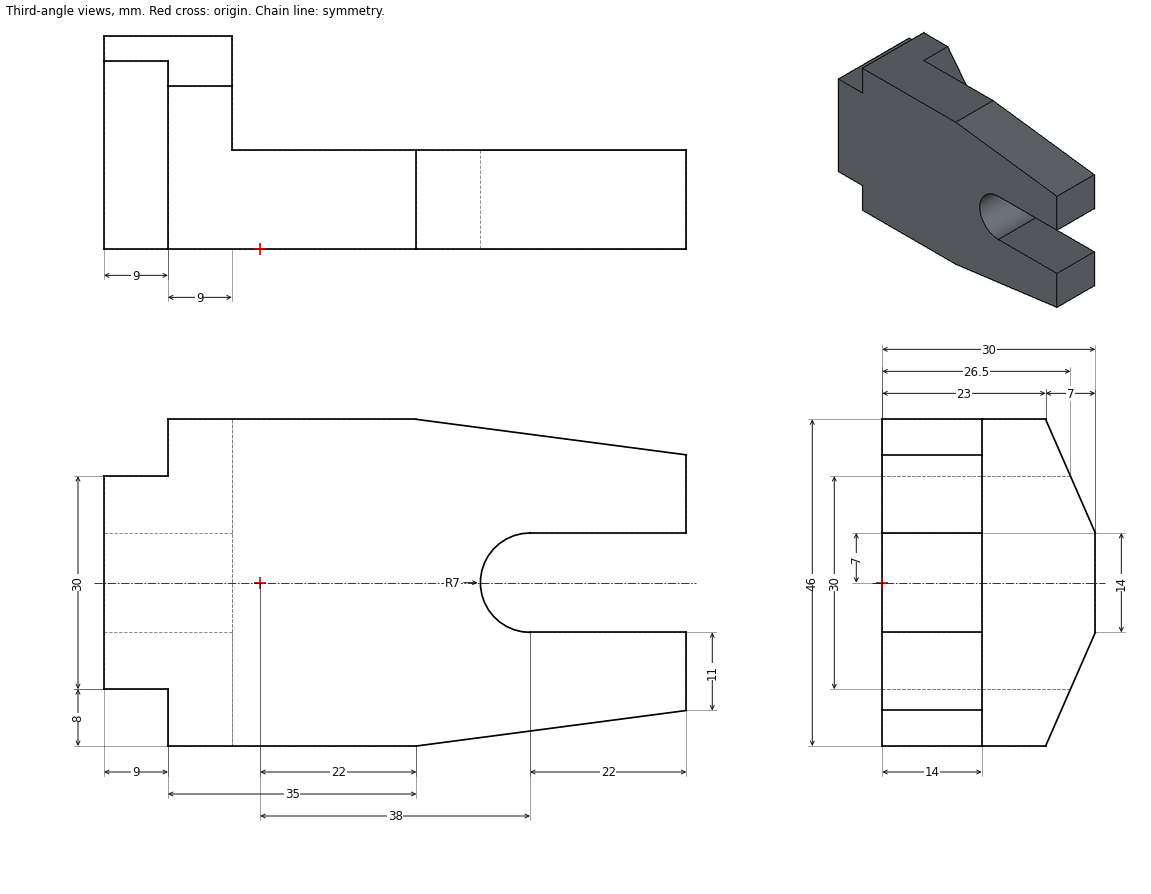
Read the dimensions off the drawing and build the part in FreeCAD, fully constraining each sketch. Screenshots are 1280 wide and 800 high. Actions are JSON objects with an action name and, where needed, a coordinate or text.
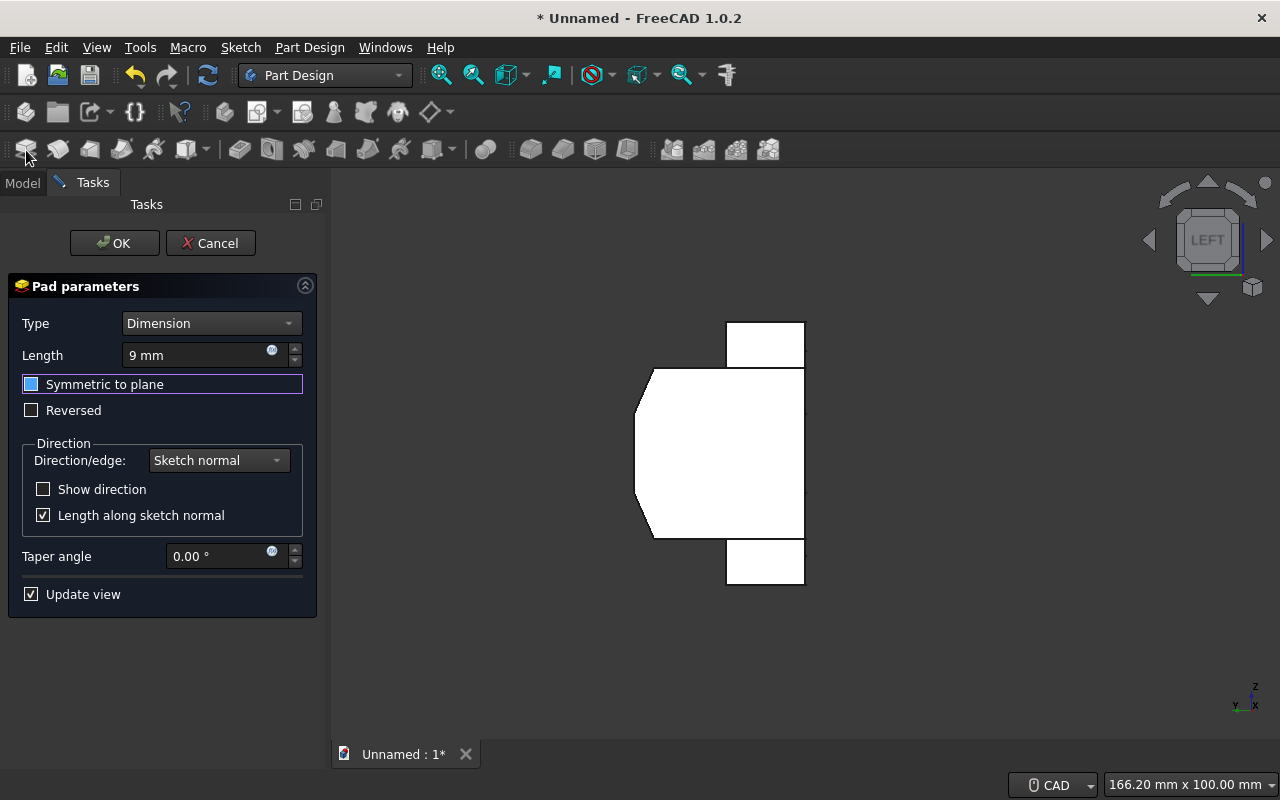
{"action": "left_click", "coordinate": [30, 410]}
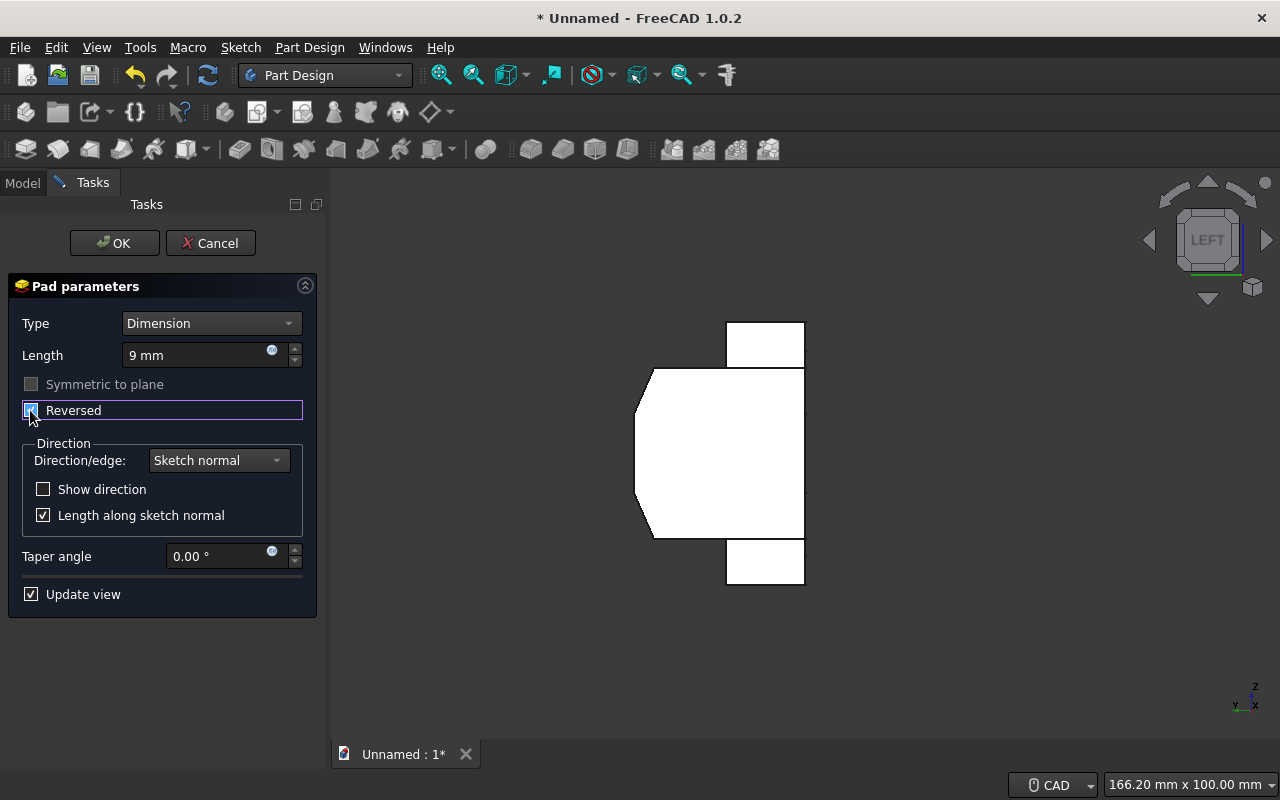
{"action": "left_click", "coordinate": [115, 243]}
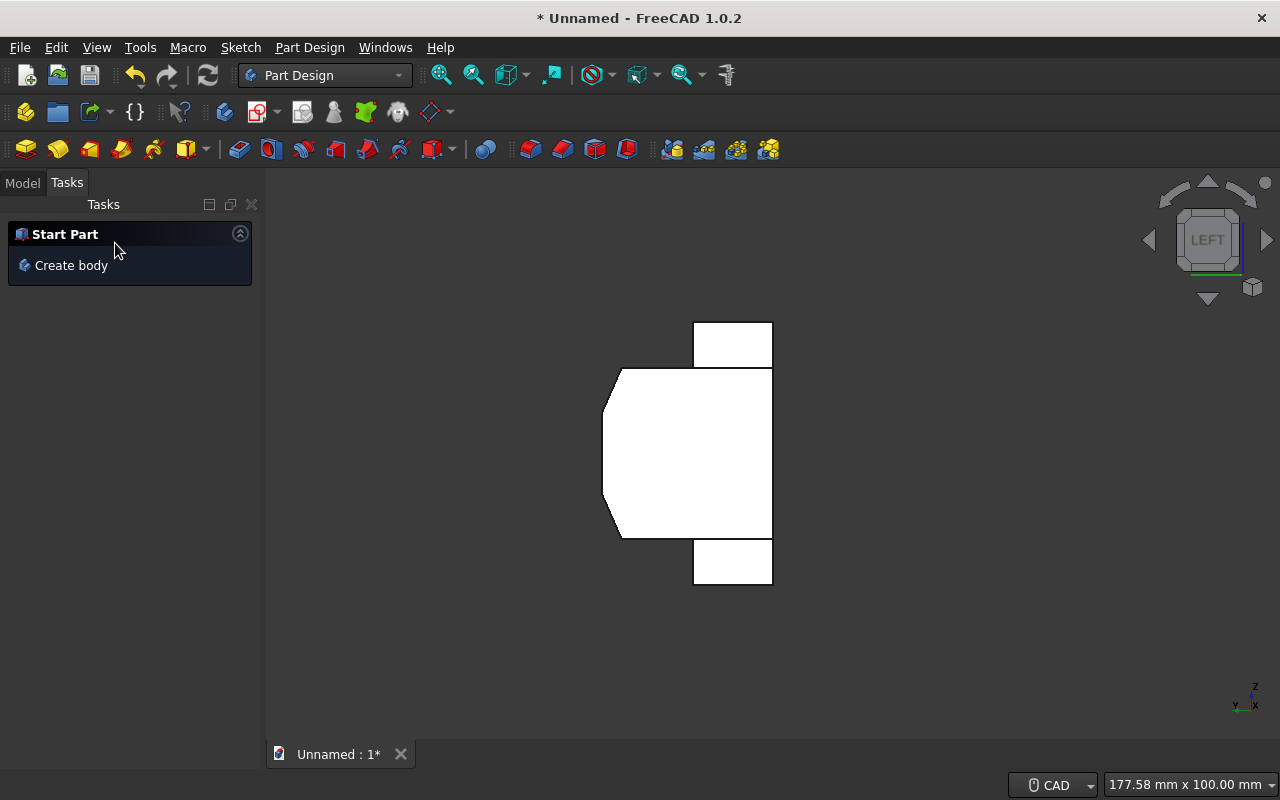
{"action": "key", "text": "0"}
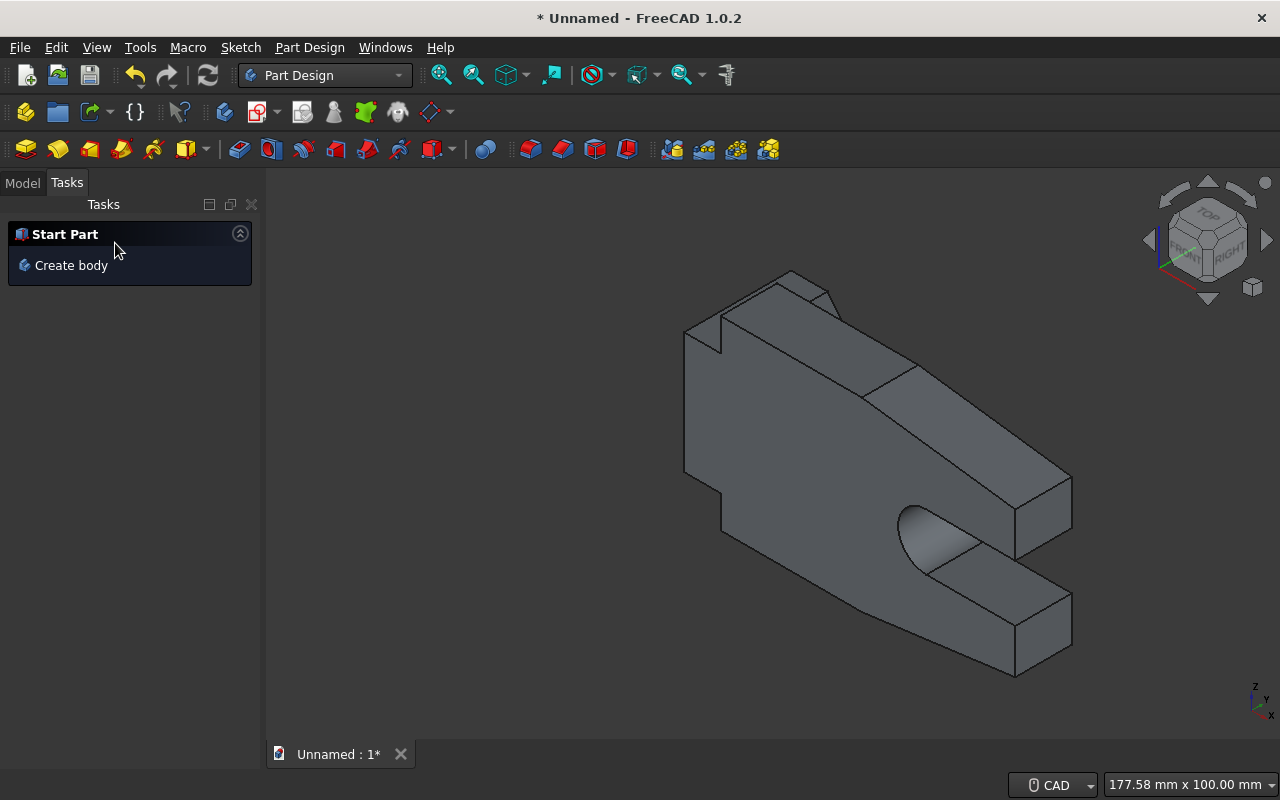
{"action": "key", "text": "3"}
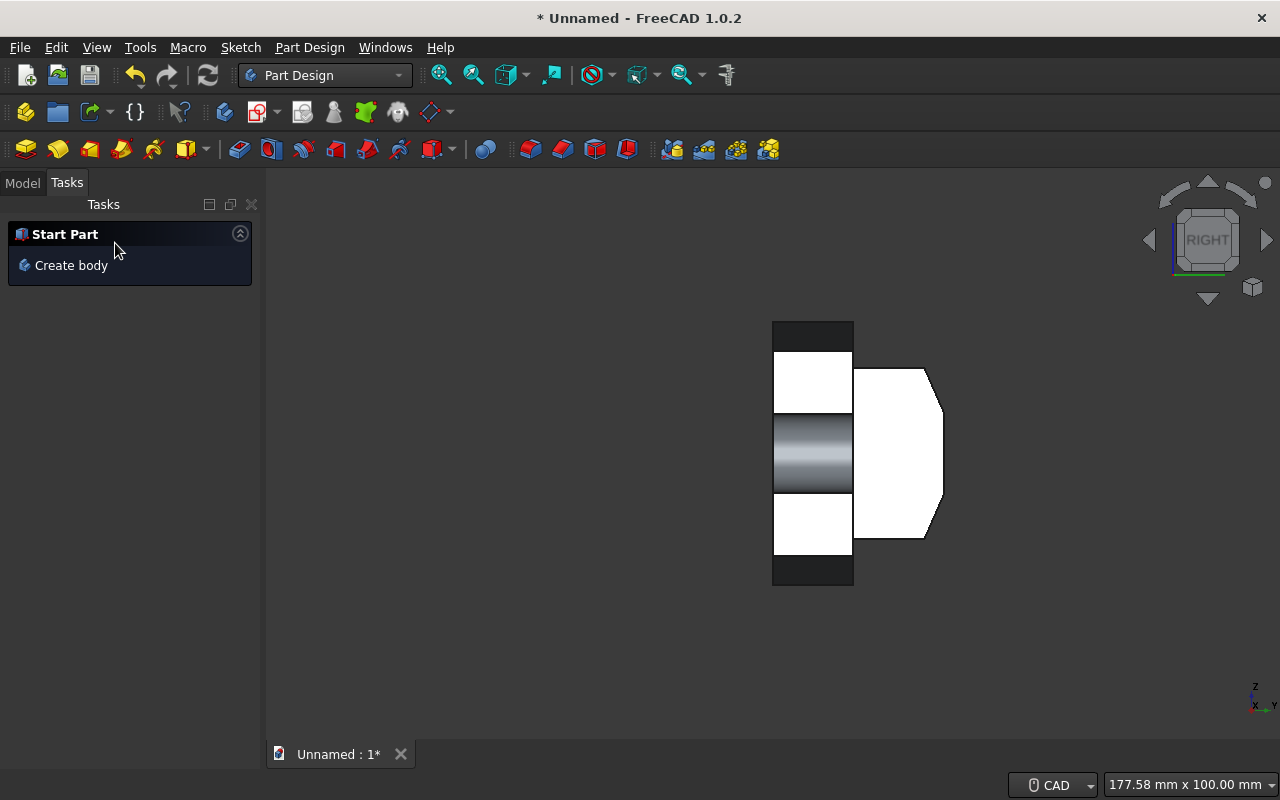
{"action": "left_click", "coordinate": [899, 428]}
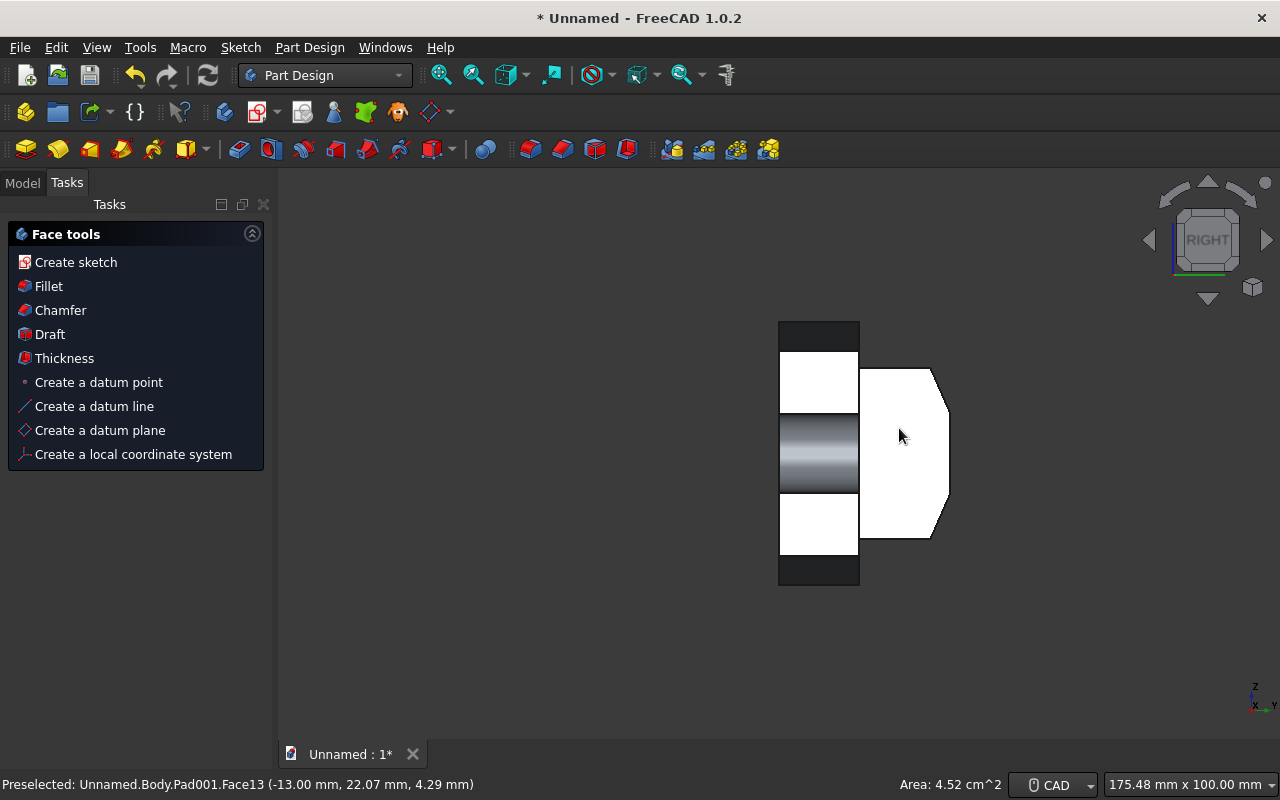
{"action": "left_click", "coordinate": [258, 112]}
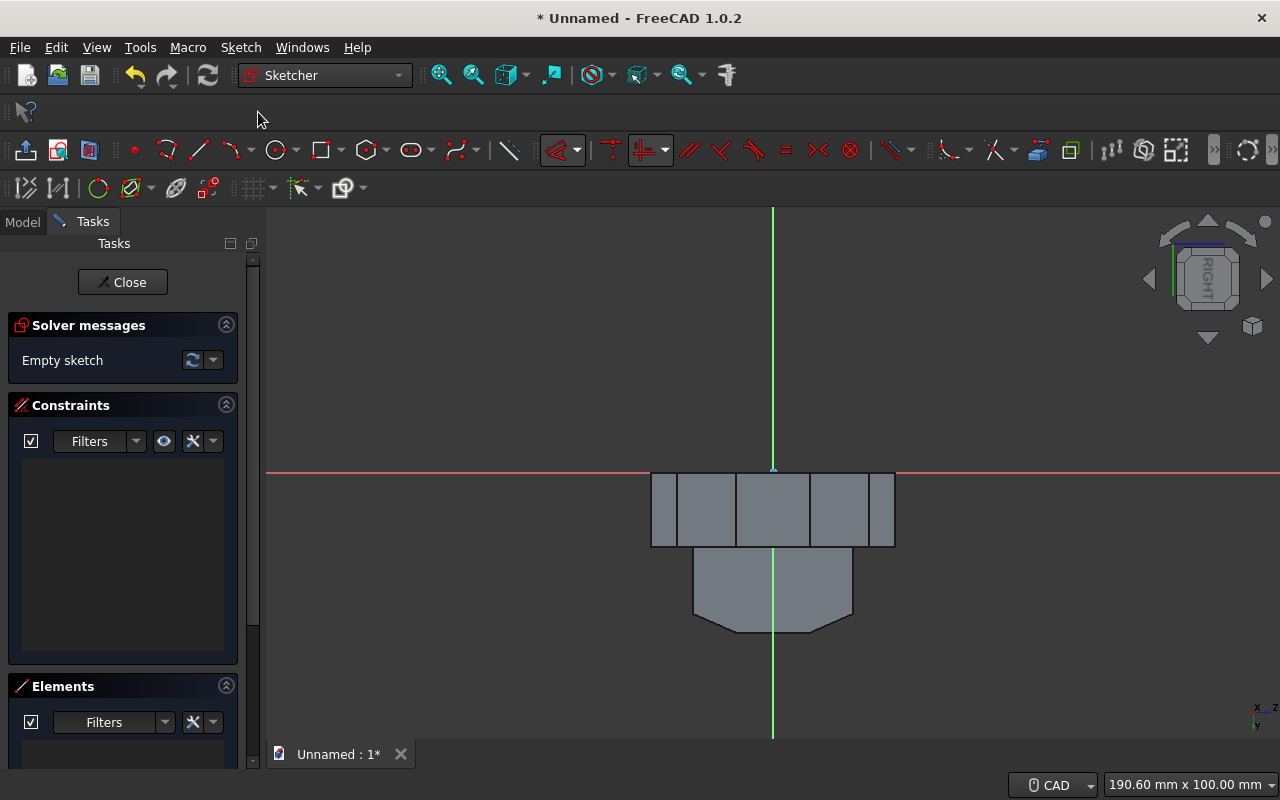
{"action": "key", "text": "q s"}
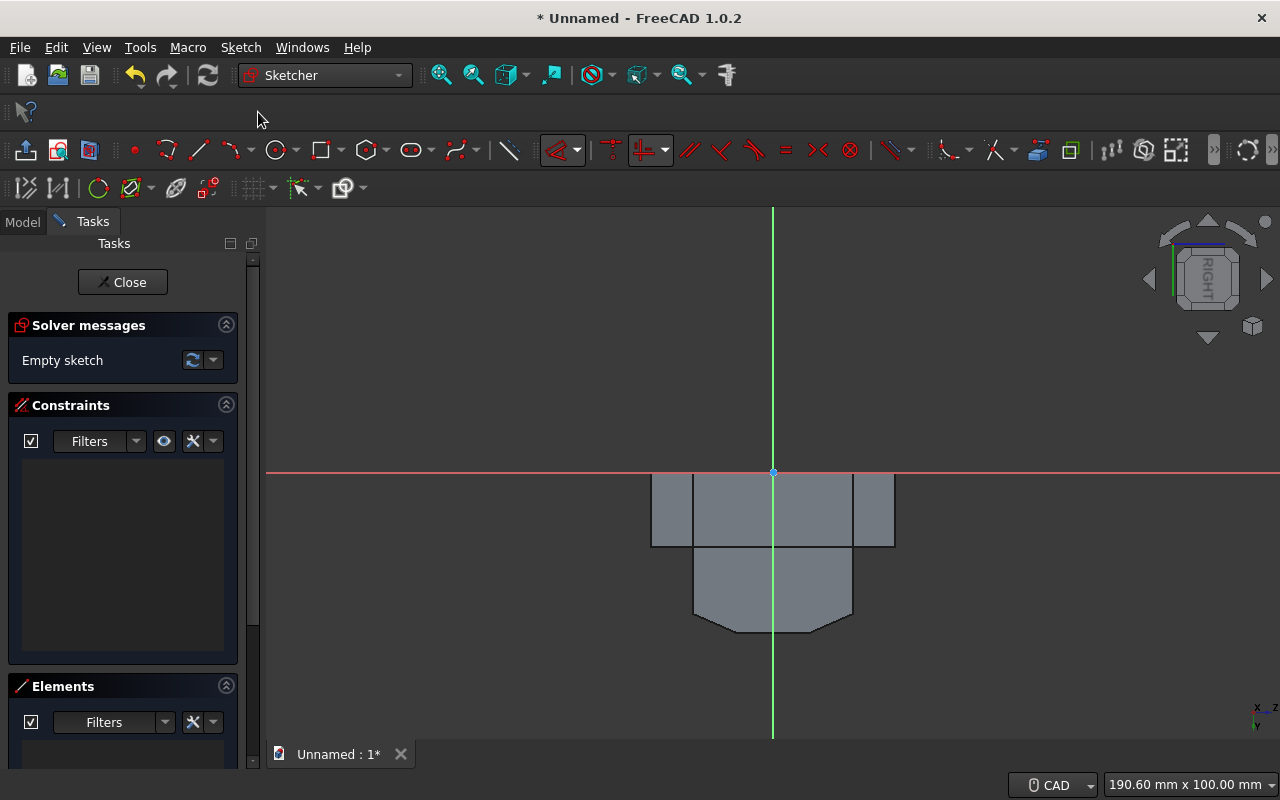
{"action": "scroll", "coordinate": [829, 618], "scroll_direction": "up", "scroll_amount": 4}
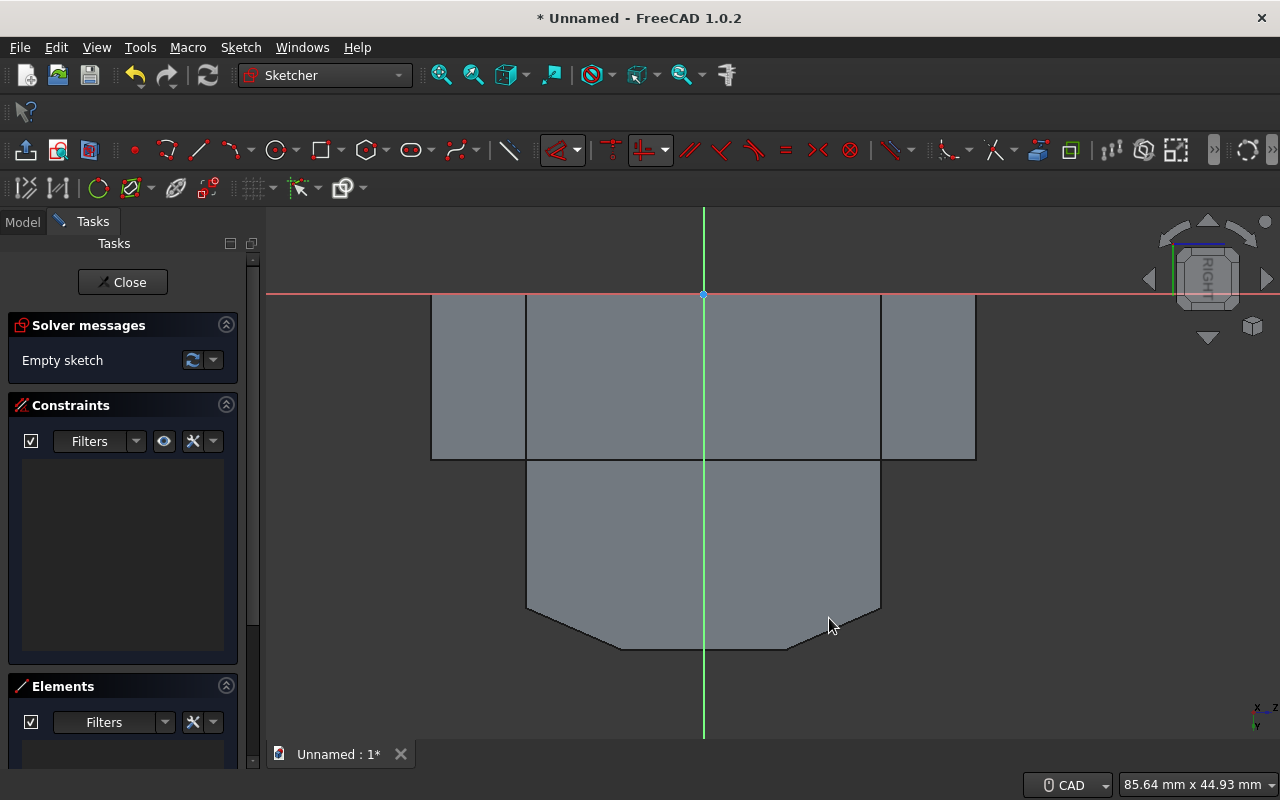
{"action": "left_click", "coordinate": [168, 150]}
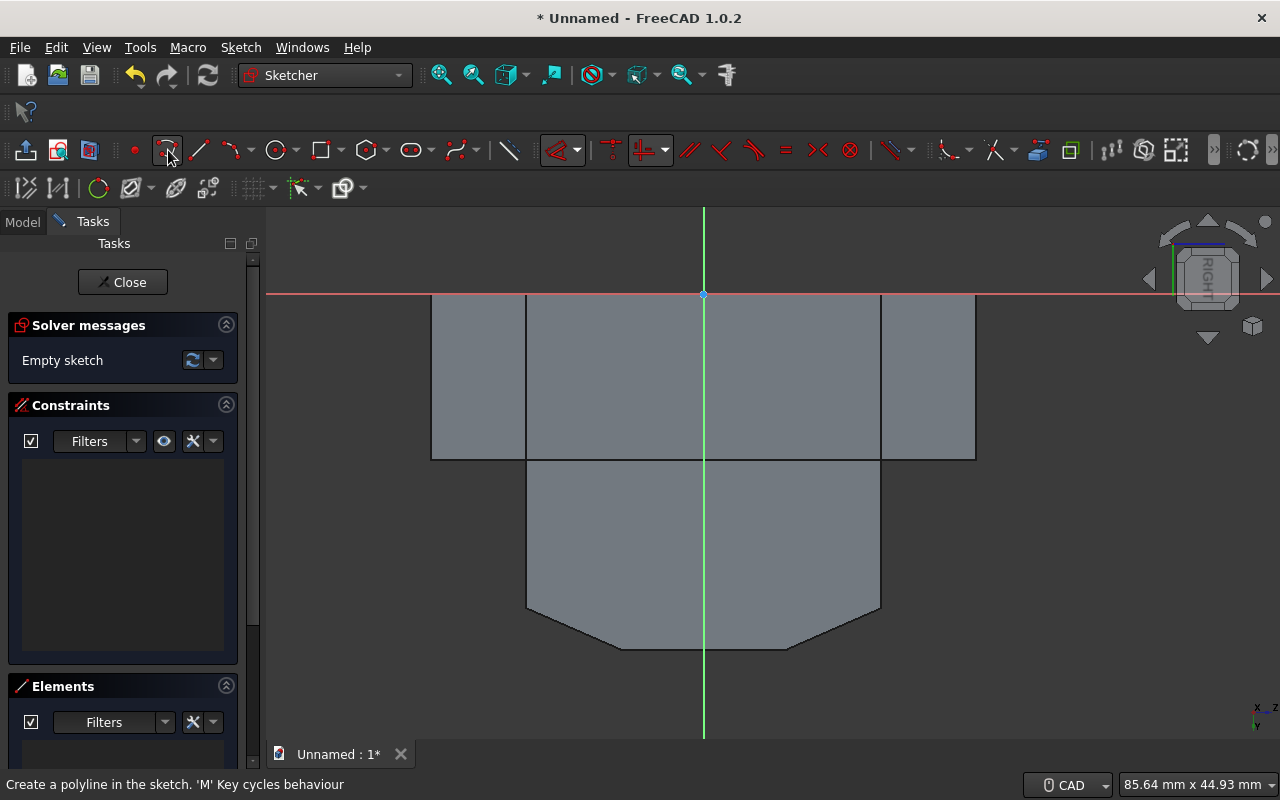
{"action": "left_click", "coordinate": [431, 294]}
{"action": "left_click", "coordinate": [976, 303]}
{"action": "left_click", "coordinate": [976, 567]}
{"action": "left_click", "coordinate": [787, 650]}
{"action": "left_click", "coordinate": [621, 650]}
{"action": "left_click", "coordinate": [431, 567]}
{"action": "left_click", "coordinate": [431, 294]}
{"action": "key", "text": "Escape"}
{"action": "key", "text": "Escape"}